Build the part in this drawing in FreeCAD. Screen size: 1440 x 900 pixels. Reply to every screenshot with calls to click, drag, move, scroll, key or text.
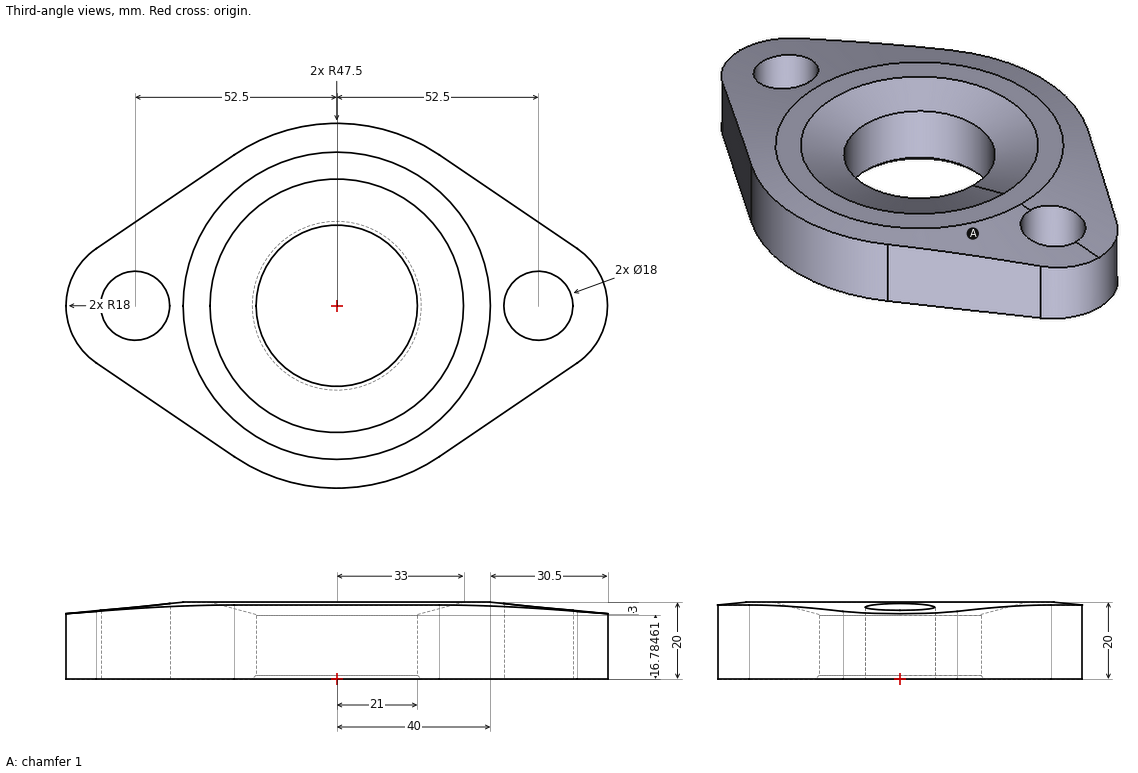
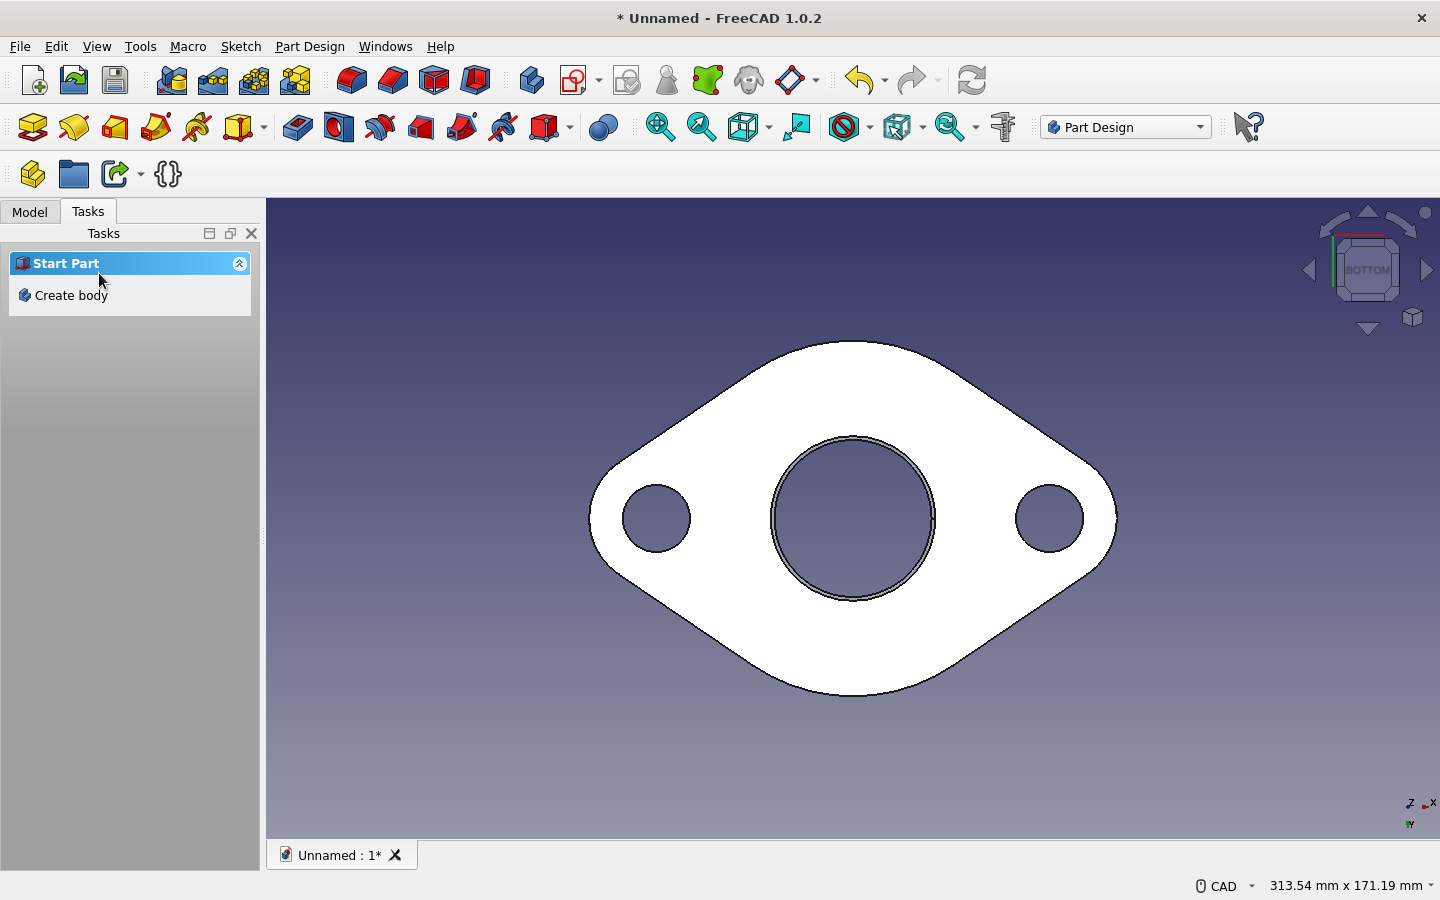
key(0)